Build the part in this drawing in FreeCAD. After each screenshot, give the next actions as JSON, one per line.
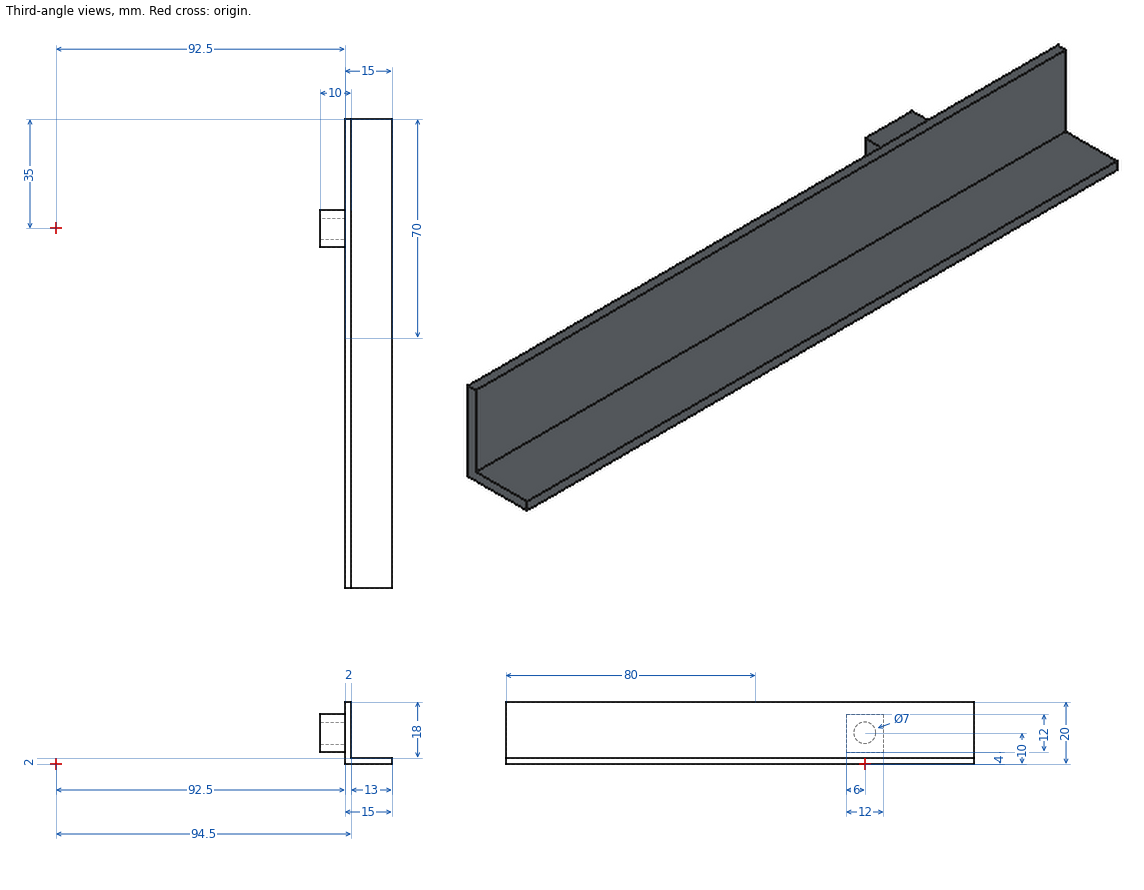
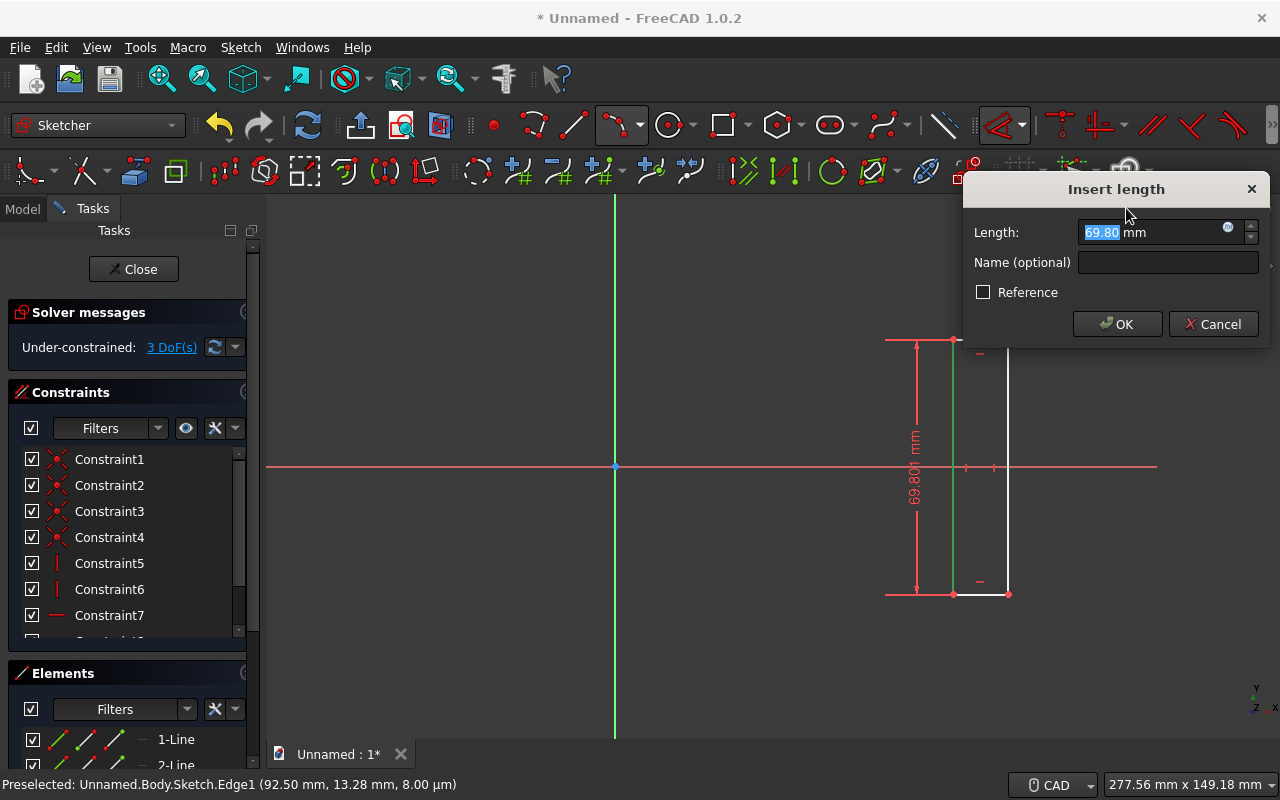
{"action": "type", "text": "70"}
{"action": "key", "text": "Return"}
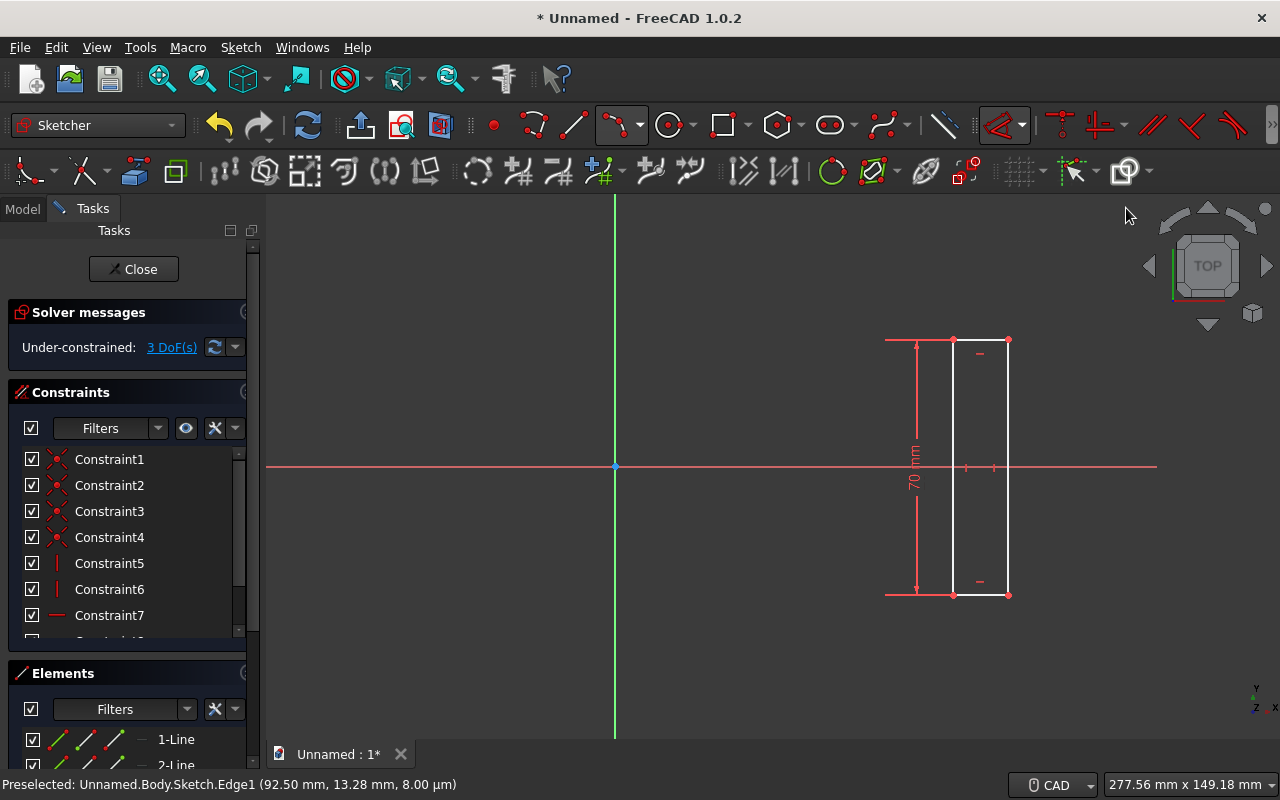
{"action": "left_click", "coordinate": [969, 595]}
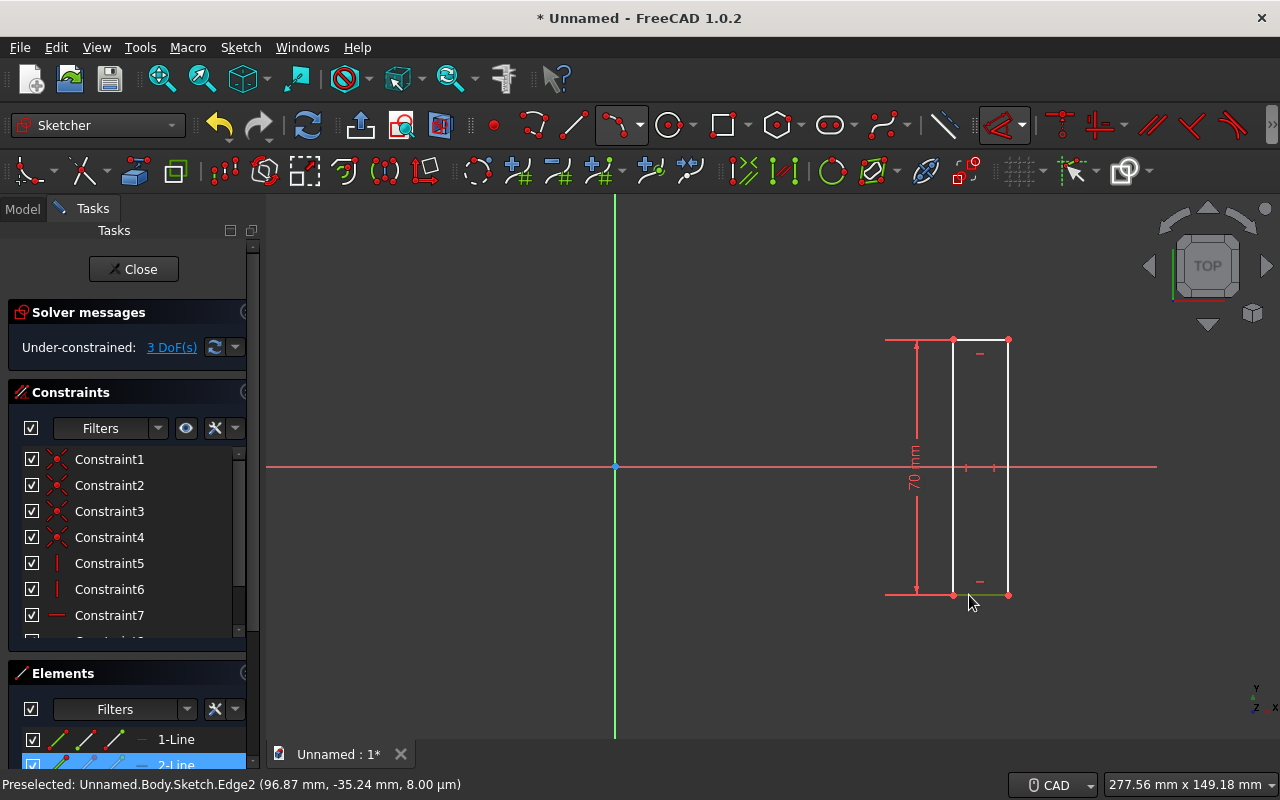
{"action": "key", "text": "l"}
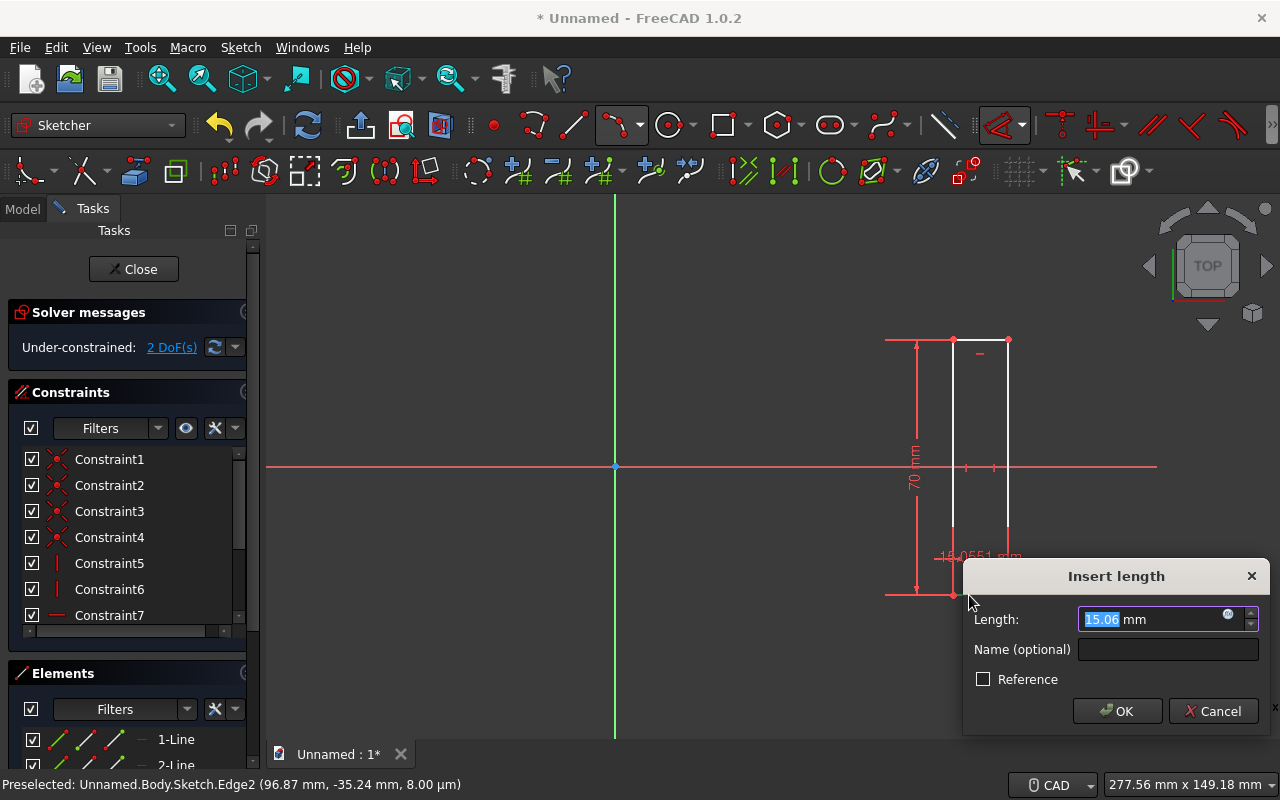
{"action": "type", "text": "15"}
{"action": "key", "text": "Return"}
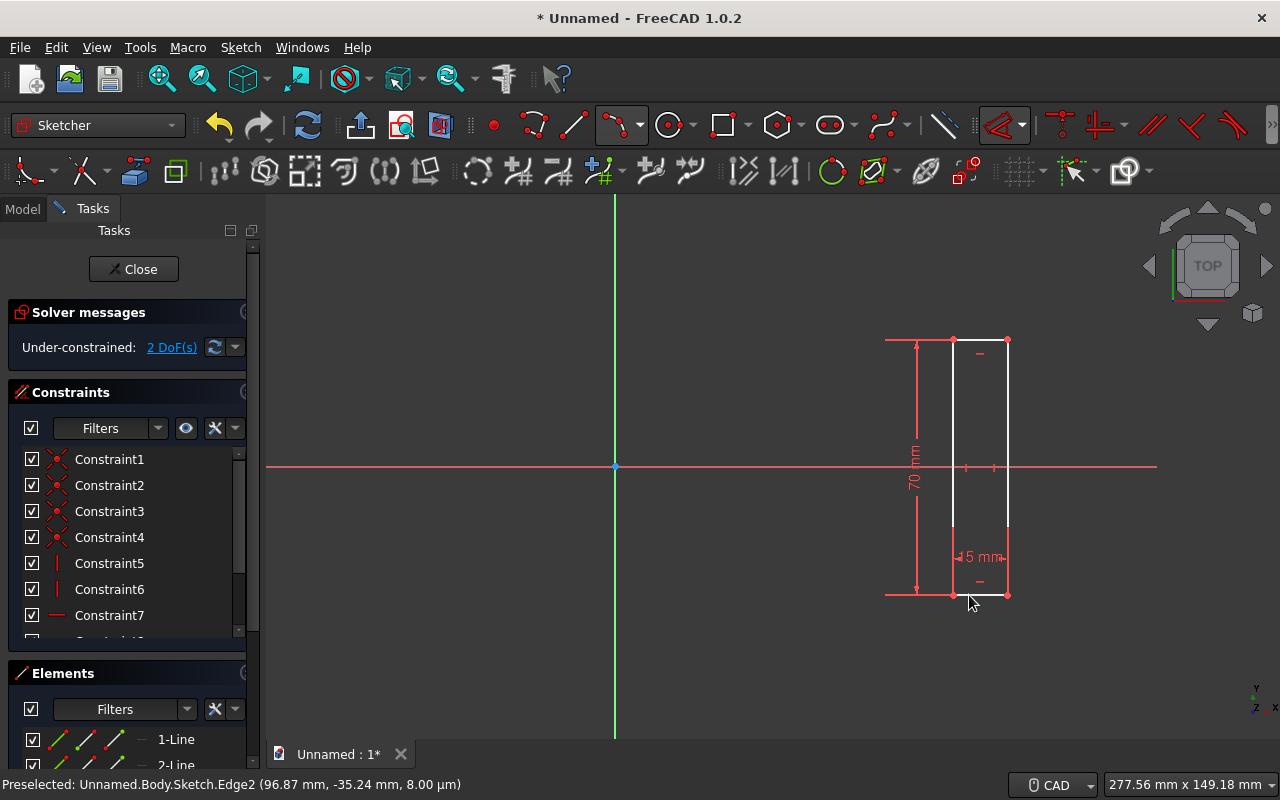
{"action": "left_click", "coordinate": [953, 340]}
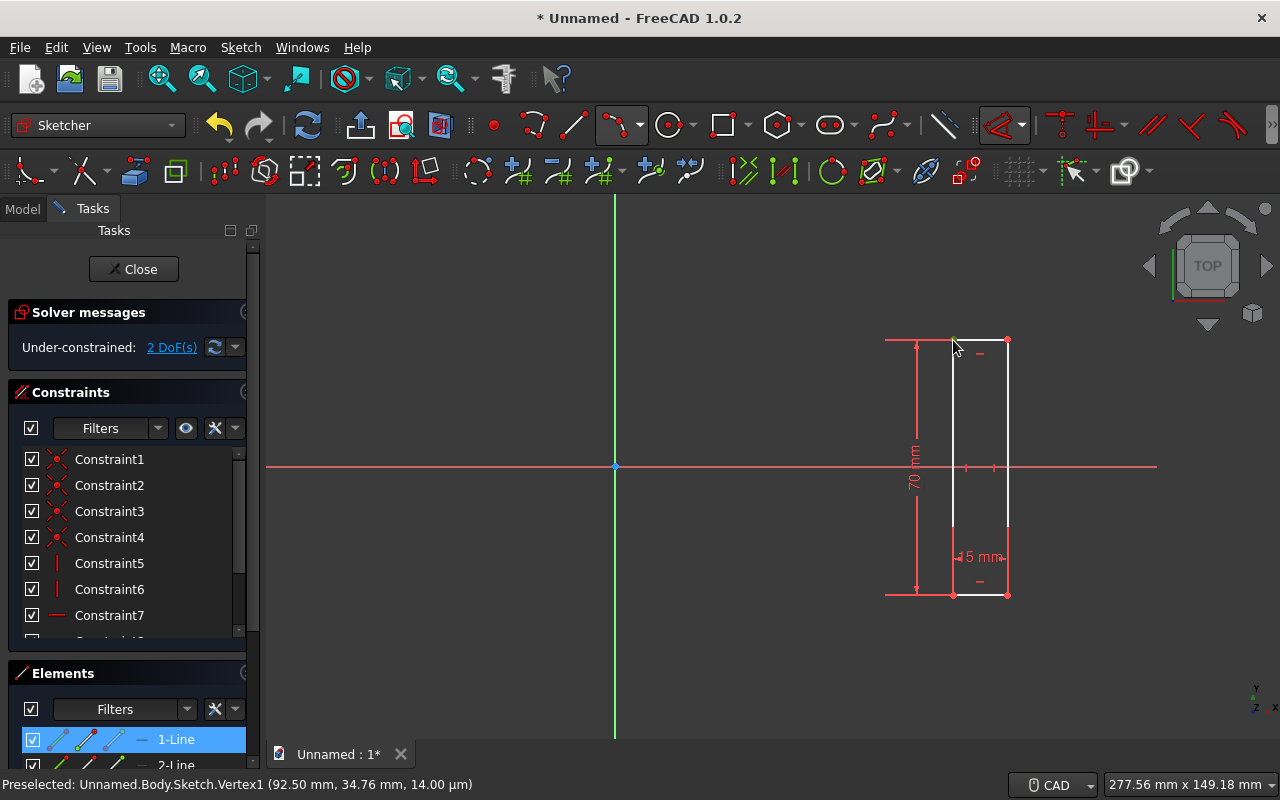
{"action": "left_click", "coordinate": [1024, 126]}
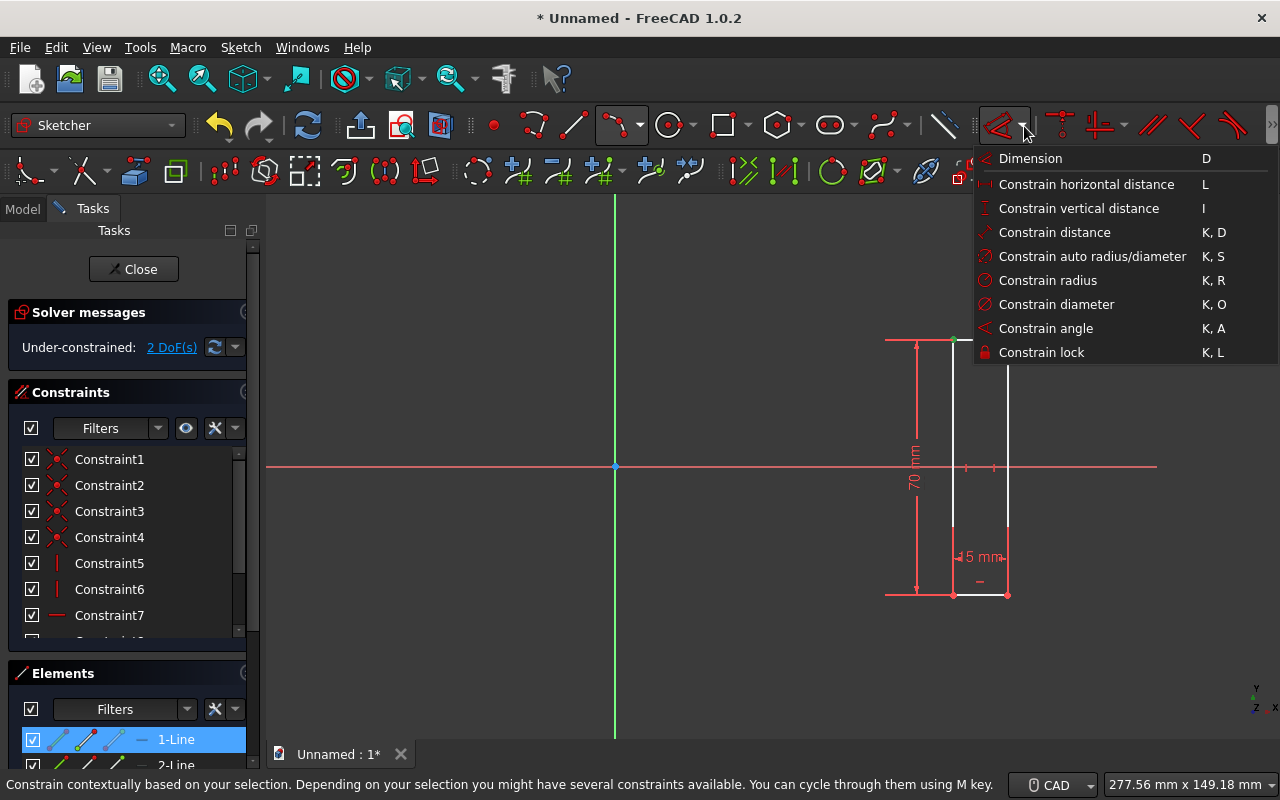
{"action": "left_click", "coordinate": [1126, 208]}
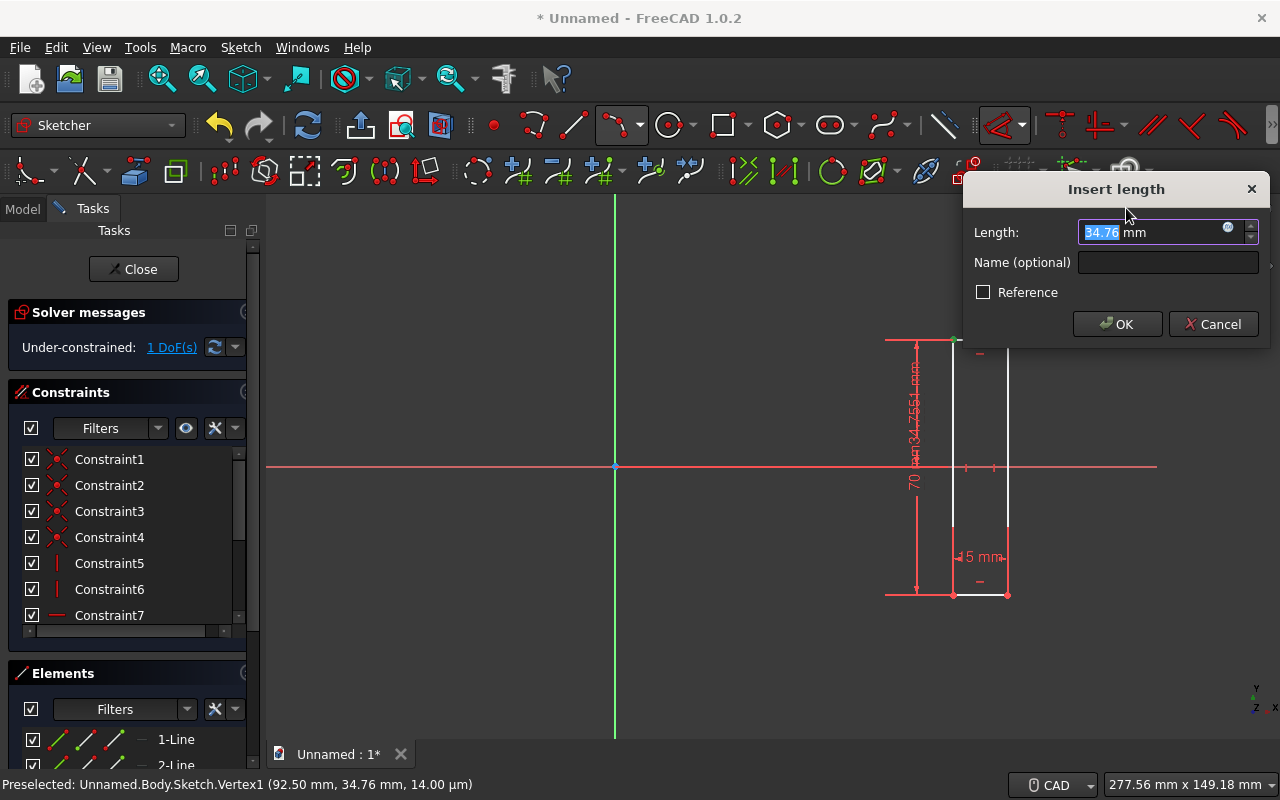
{"action": "type", "text": "35"}
{"action": "key", "text": "Return"}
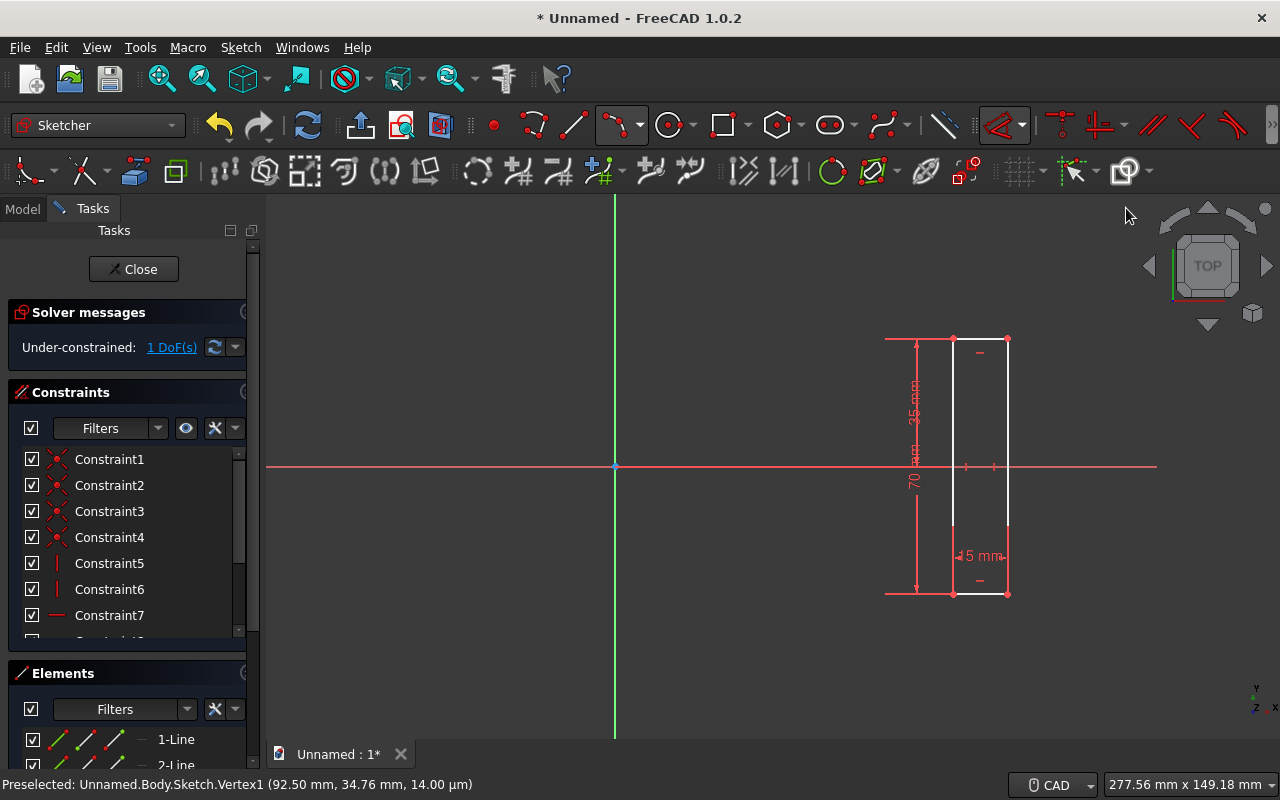
{"action": "left_click", "coordinate": [953, 339]}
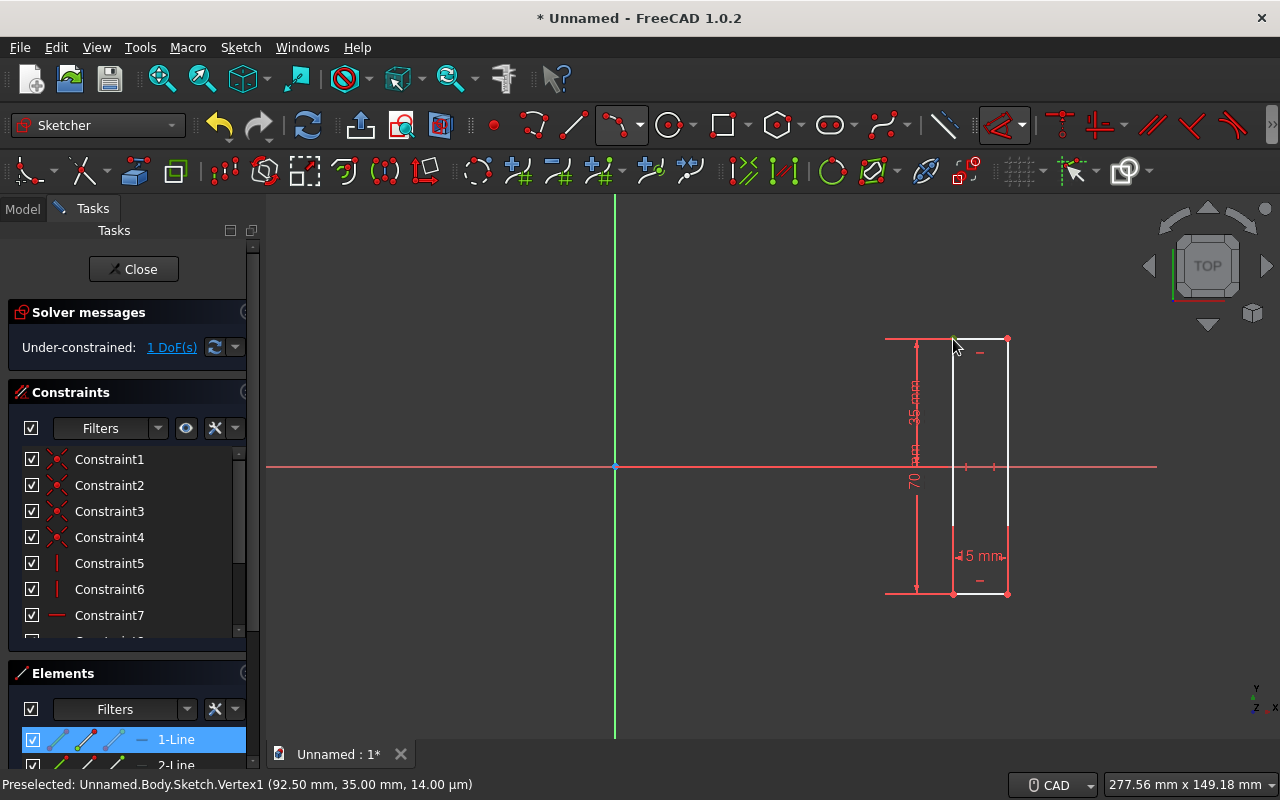
{"action": "key", "text": "l"}